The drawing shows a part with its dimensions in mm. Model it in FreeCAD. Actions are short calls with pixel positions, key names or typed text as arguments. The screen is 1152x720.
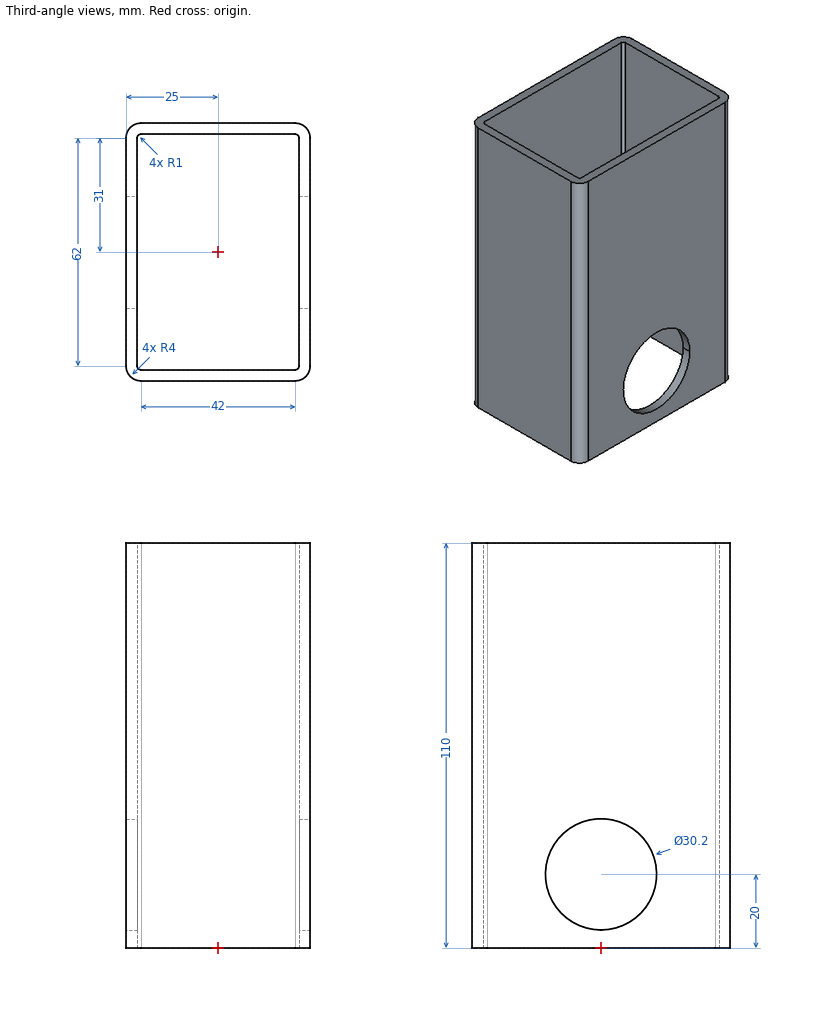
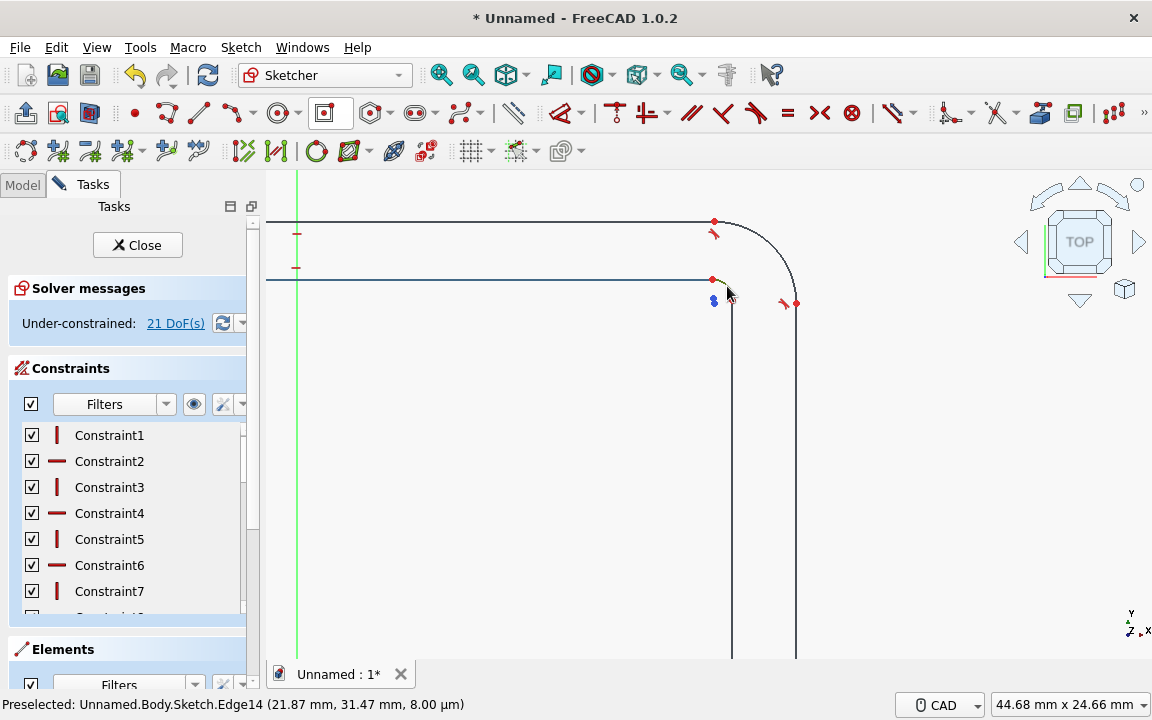
click(756, 114)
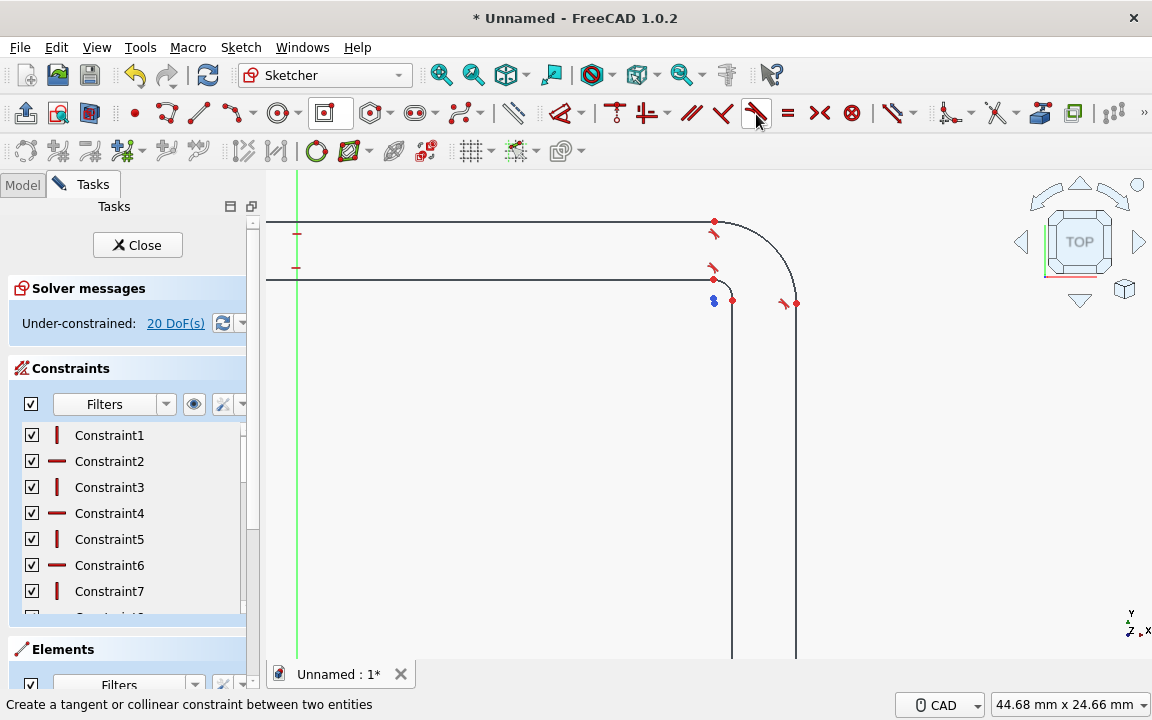
scroll(727, 288, down, 8)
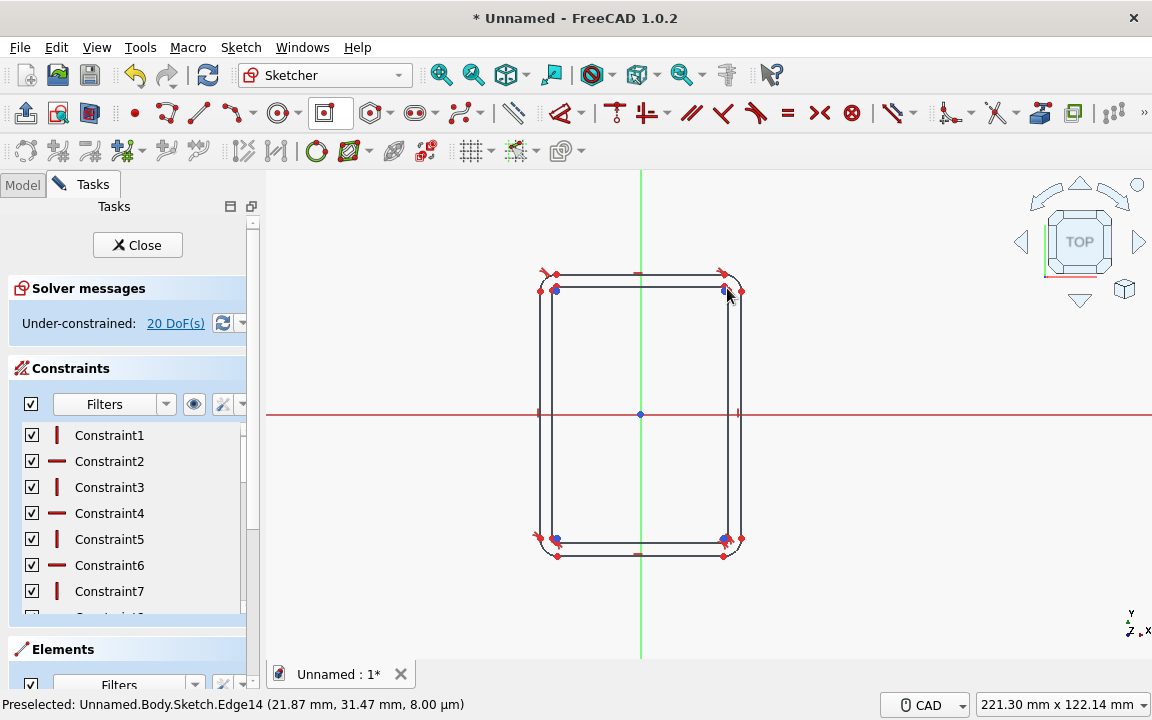
click(728, 340)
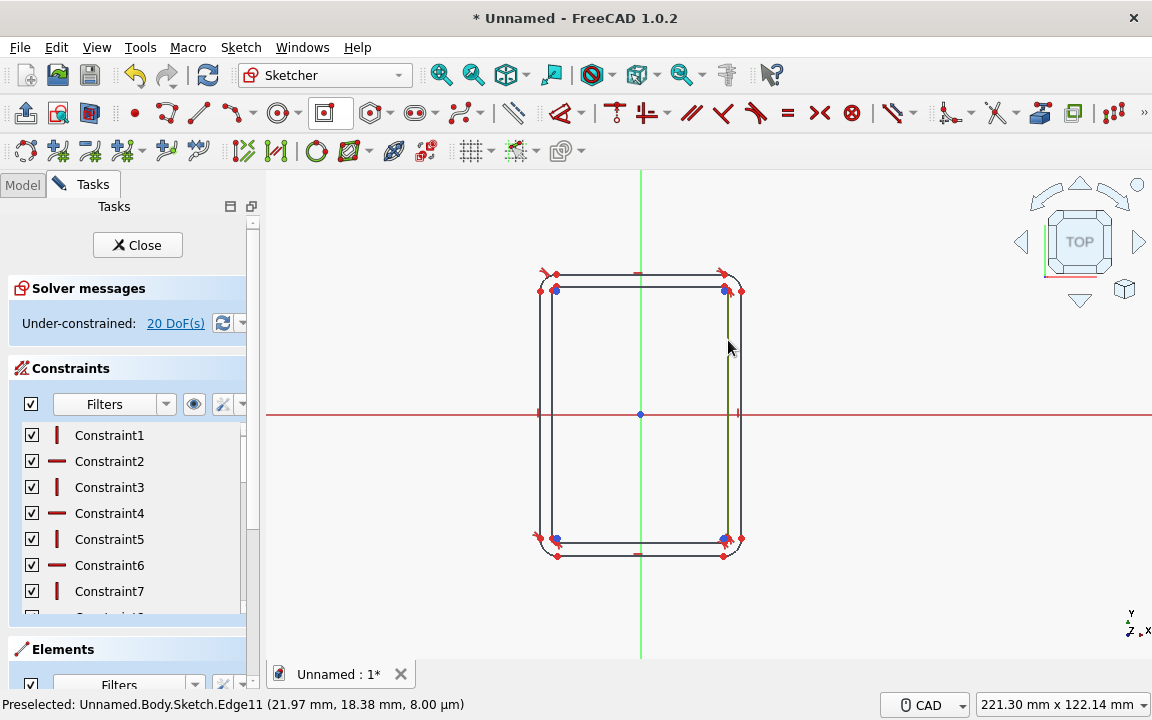
scroll(728, 288, up, 8)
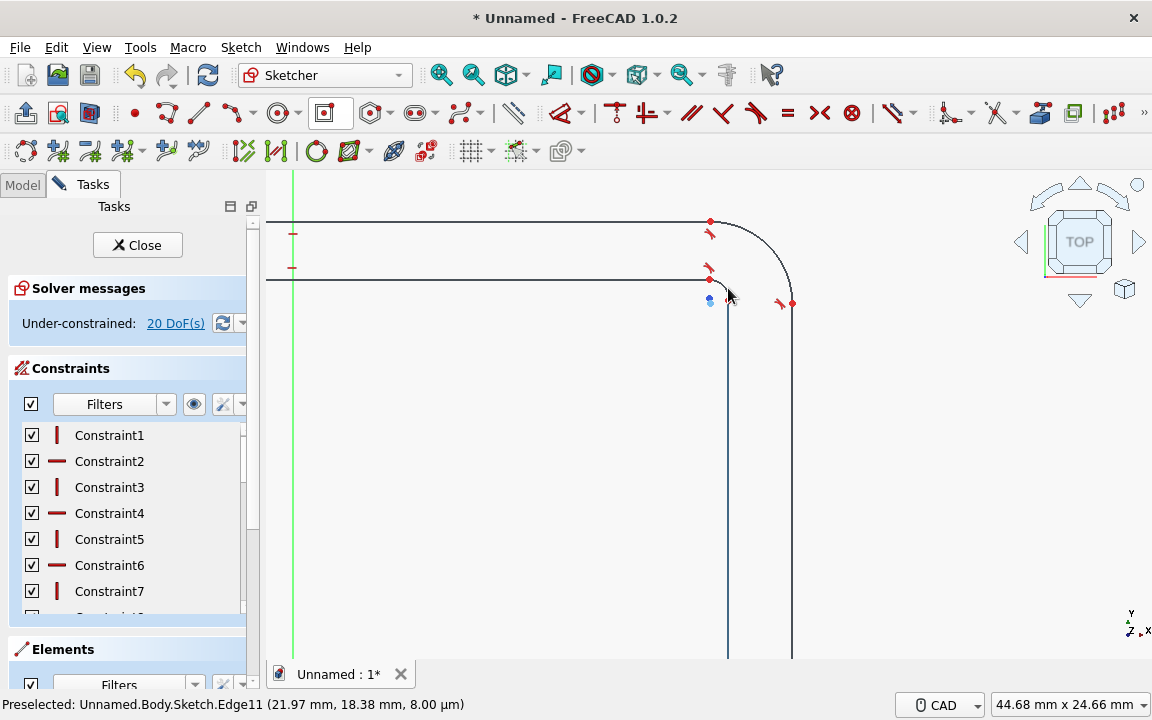
click(724, 286)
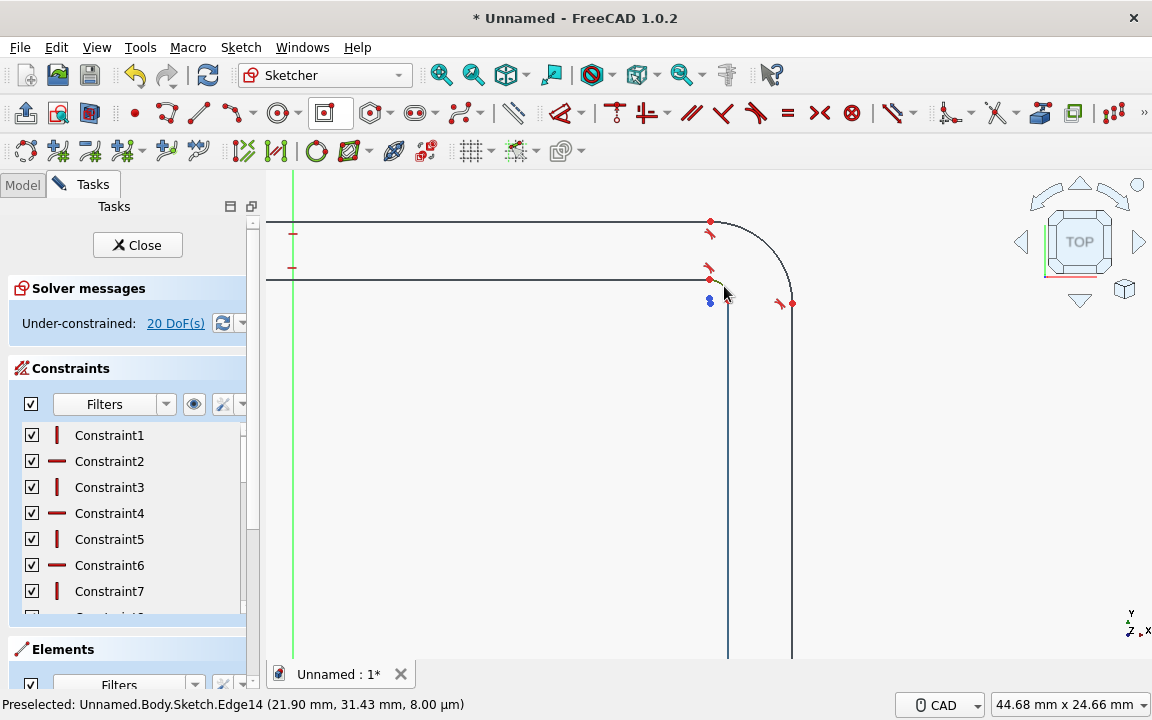
key(t)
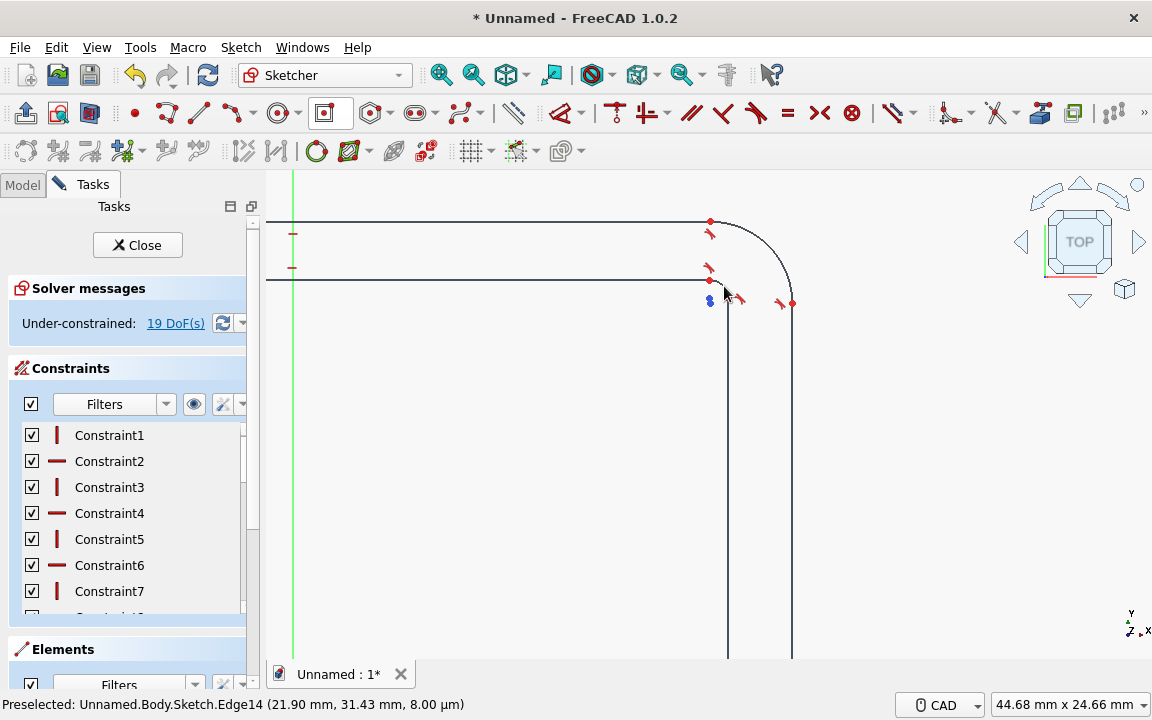
scroll(728, 288, down, 8)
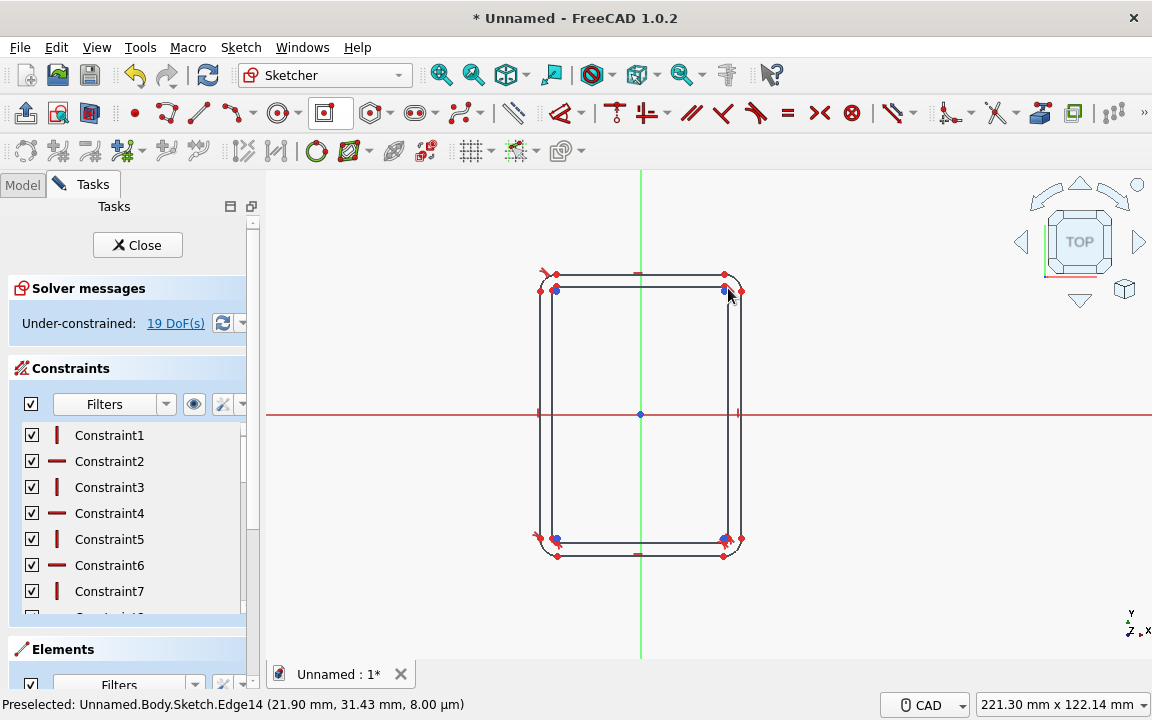
click(728, 340)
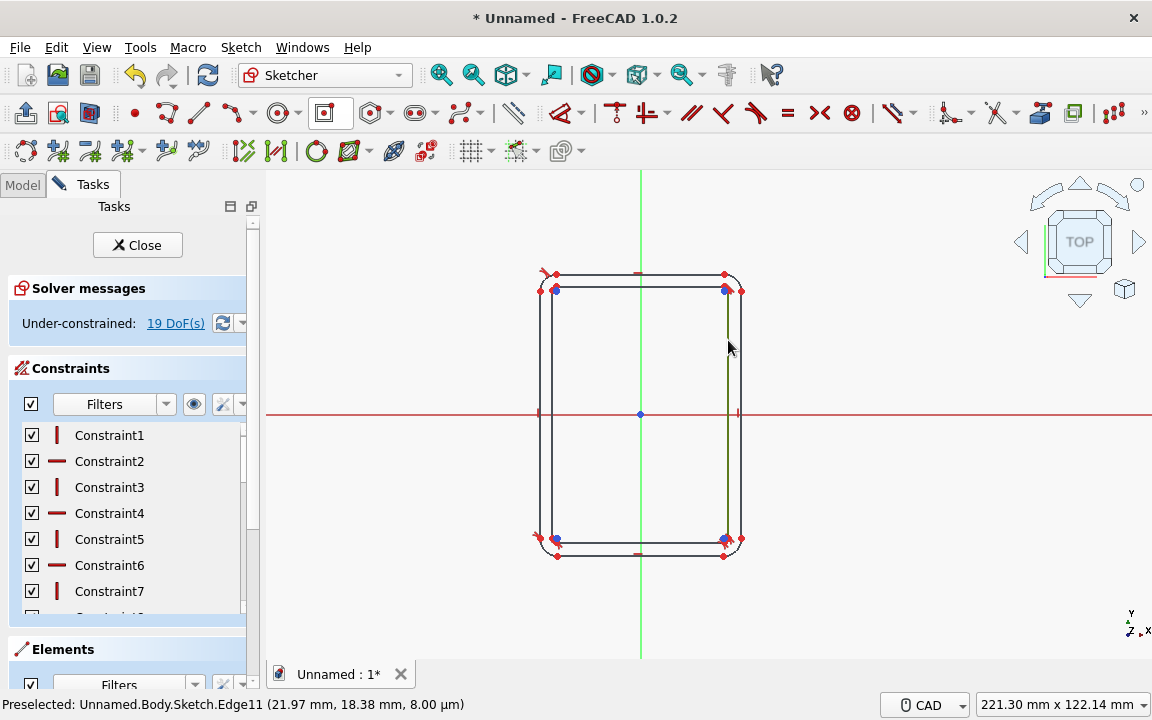
scroll(727, 542, up, 8)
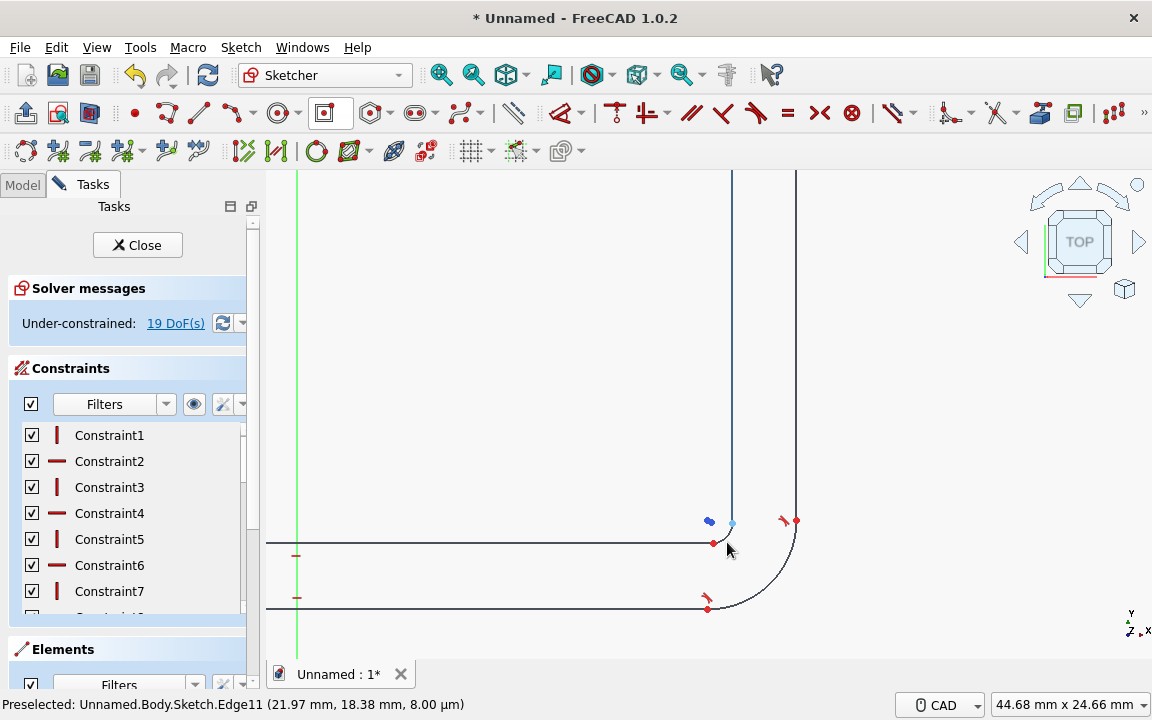
click(726, 537)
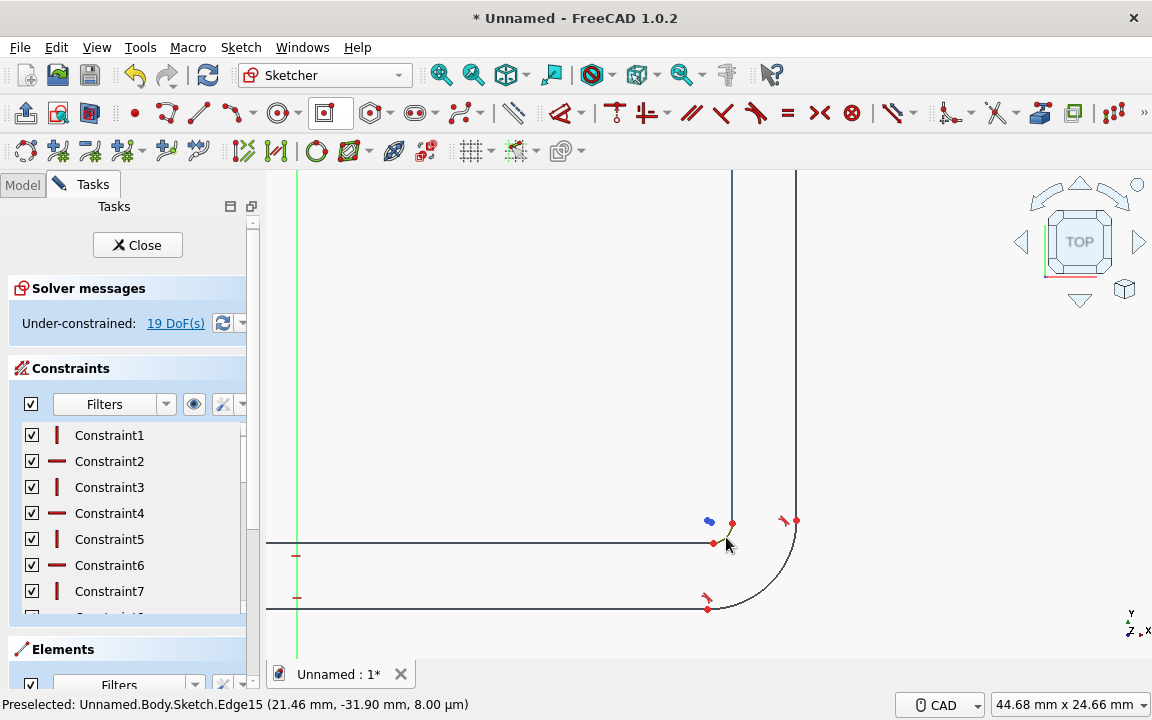
key(t)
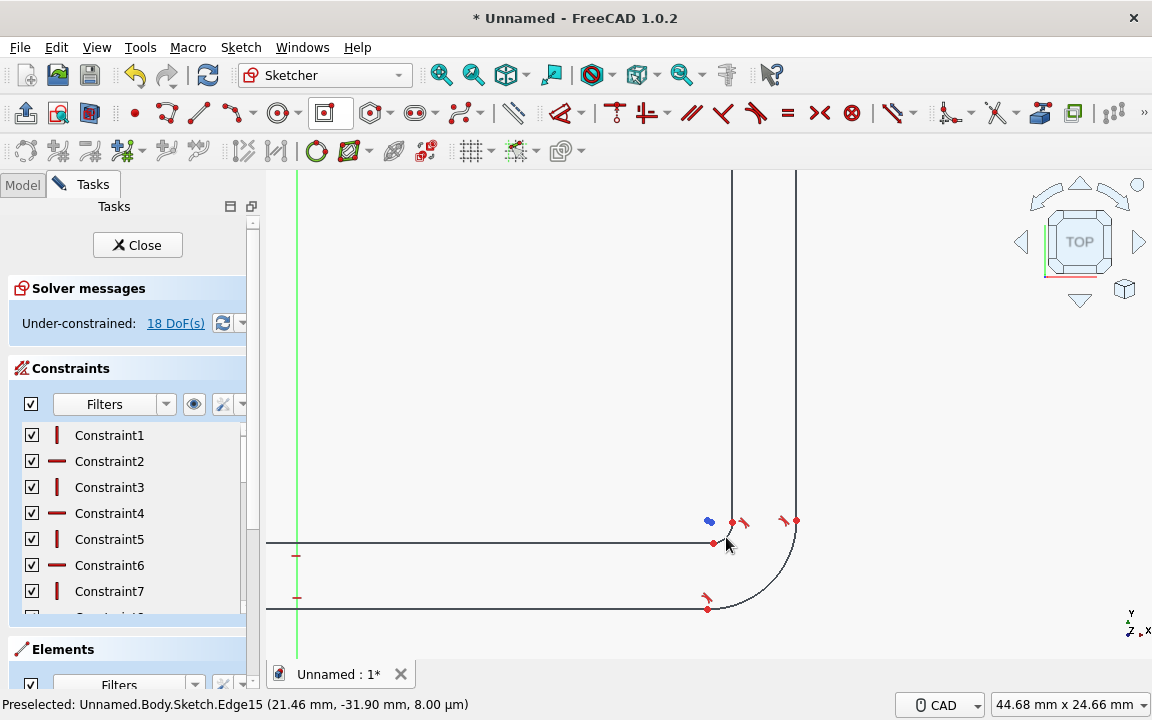
scroll(727, 543, down, 8)